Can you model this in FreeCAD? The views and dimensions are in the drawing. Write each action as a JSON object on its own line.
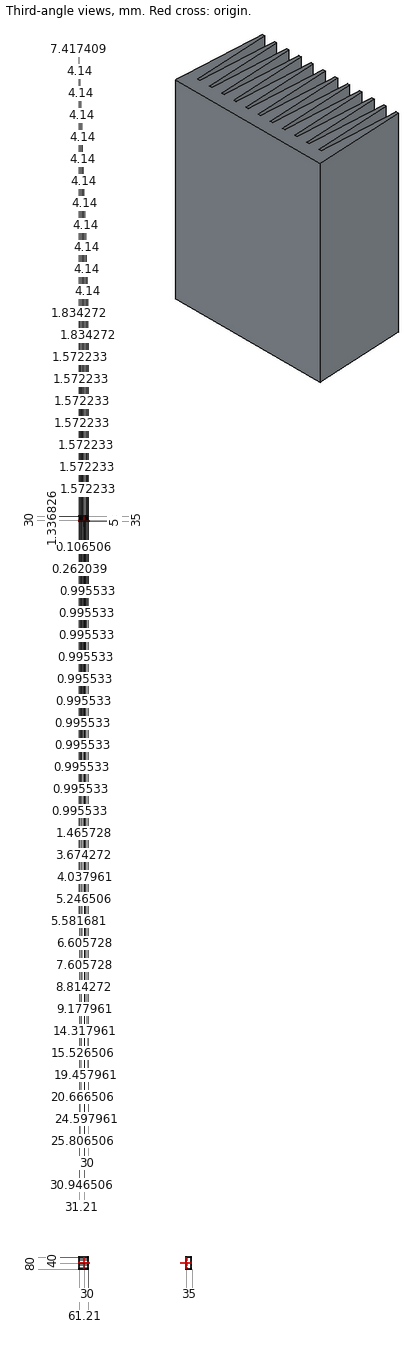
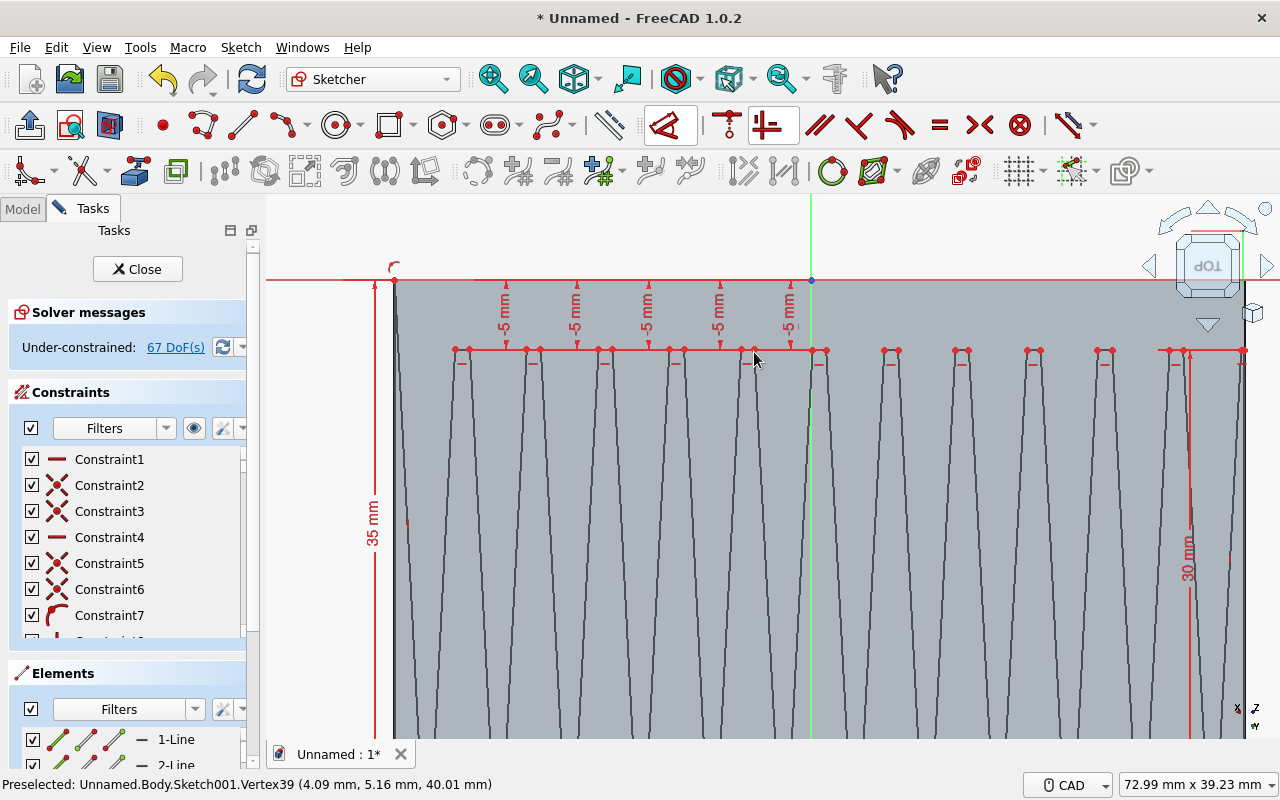
{"action": "left_click", "coordinate": [813, 350]}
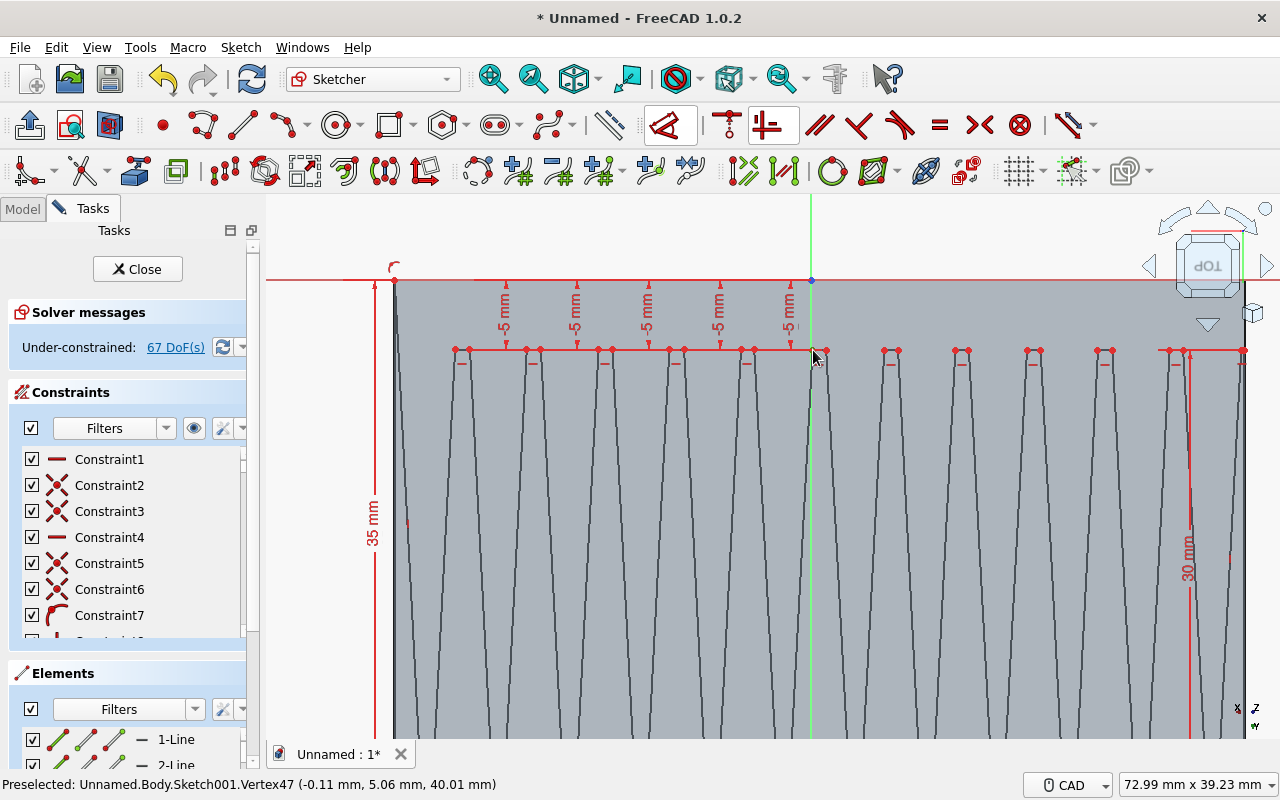
{"action": "left_click", "coordinate": [692, 126]}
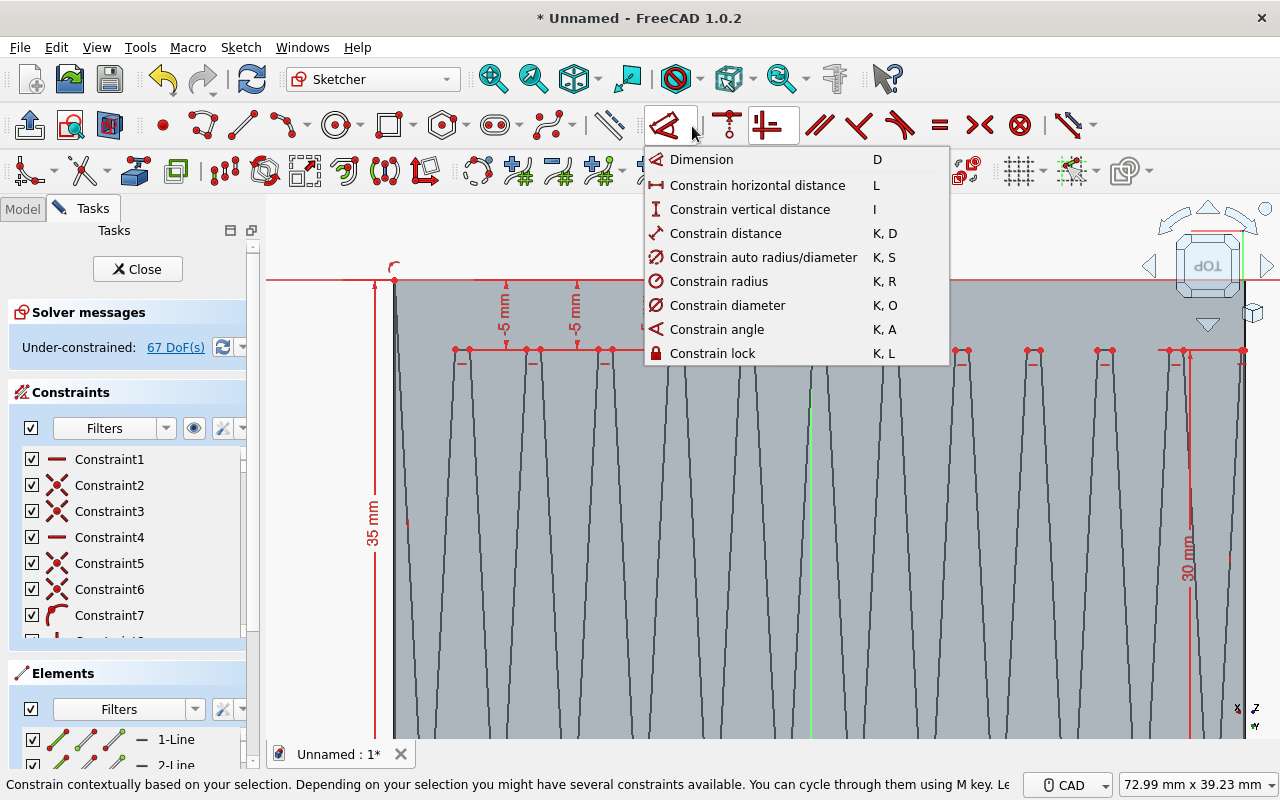
{"action": "left_click", "coordinate": [797, 209]}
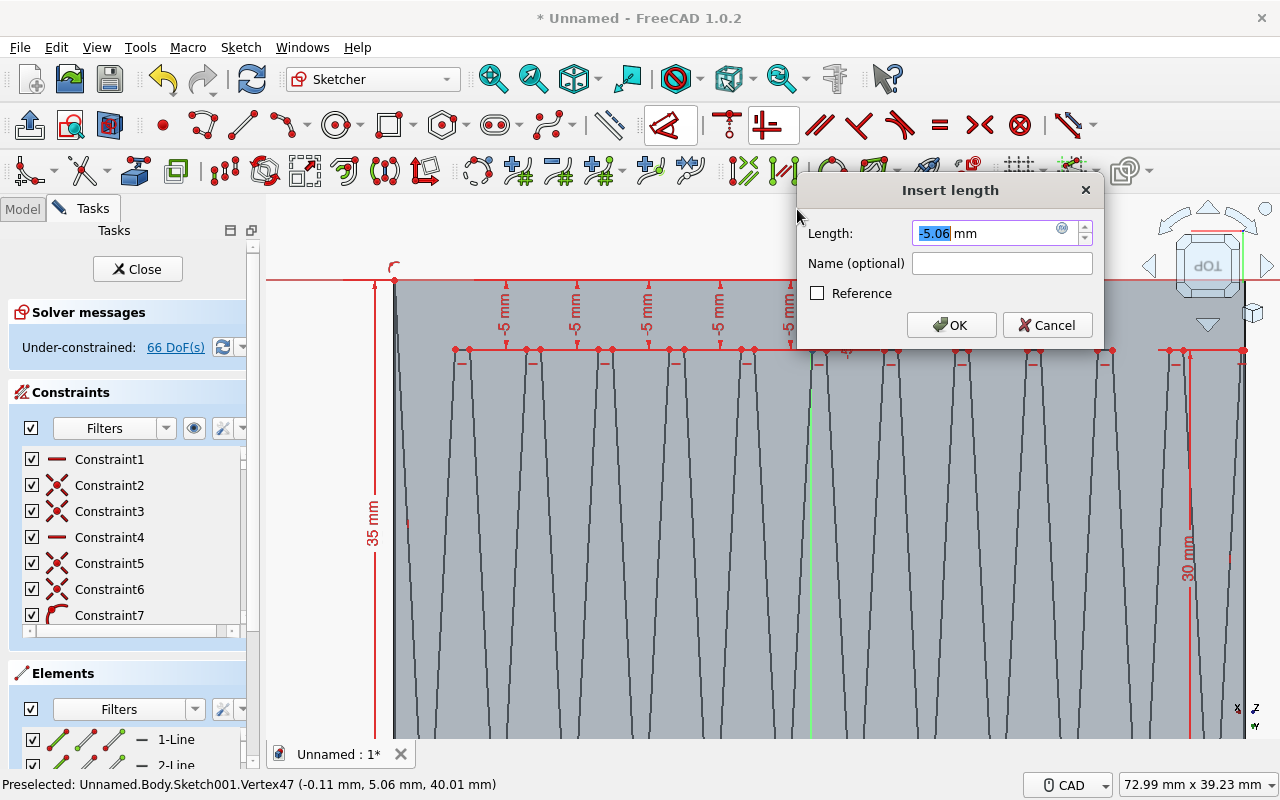
{"action": "type", "text": "-5"}
{"action": "key", "text": "Return"}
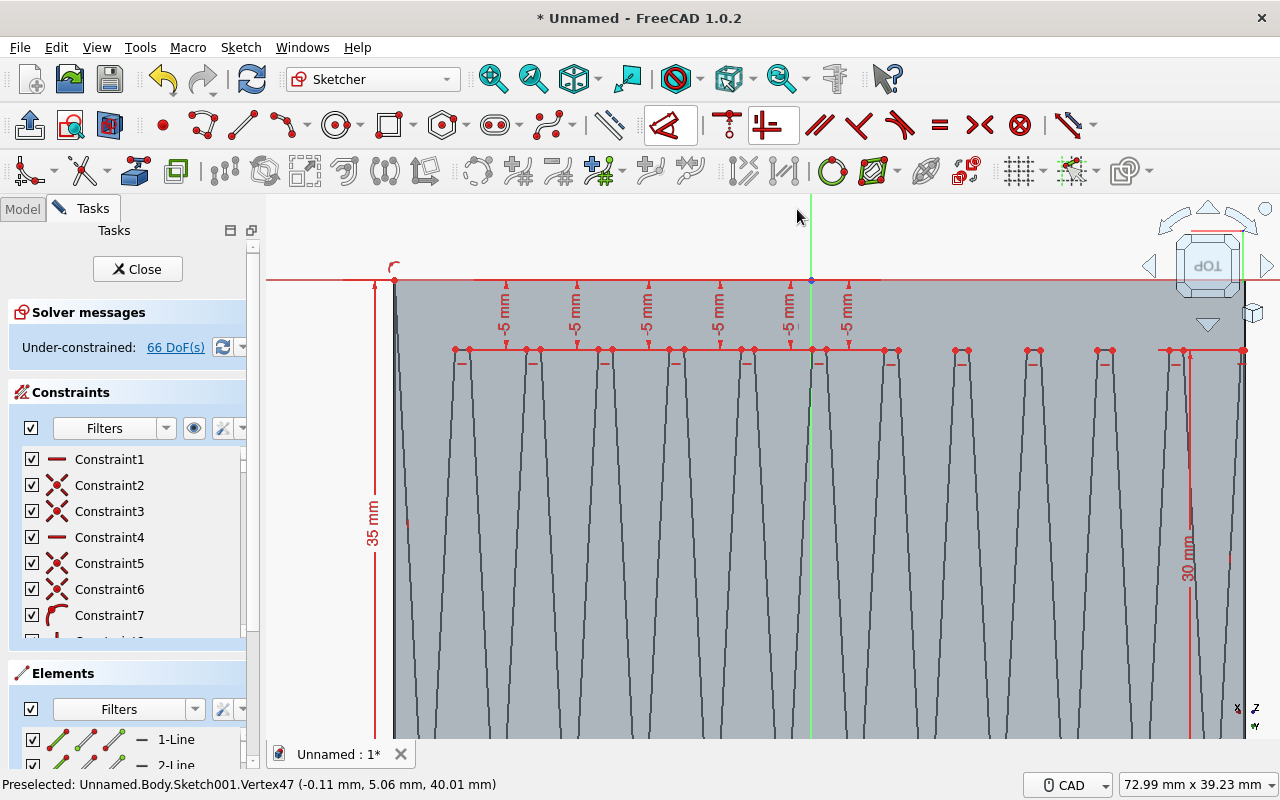
{"action": "left_click", "coordinate": [884, 350]}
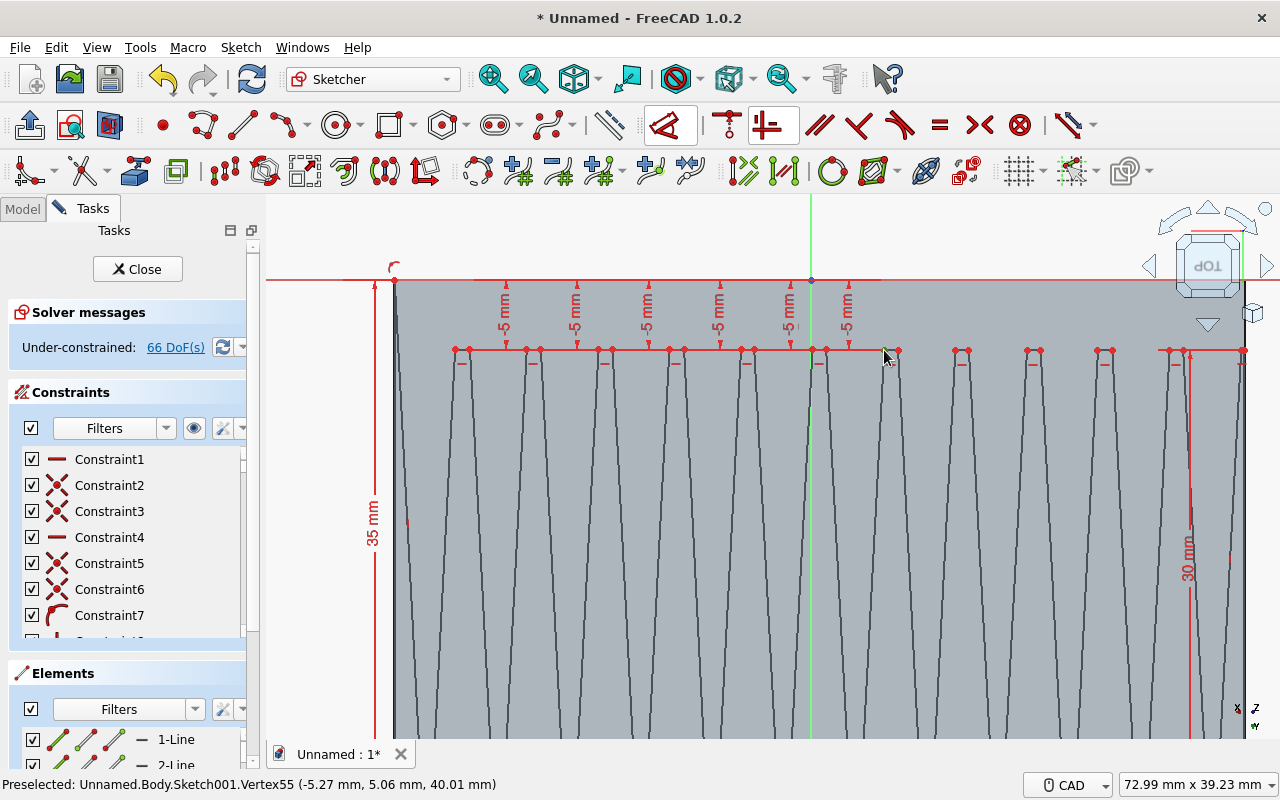
{"action": "key", "text": "i"}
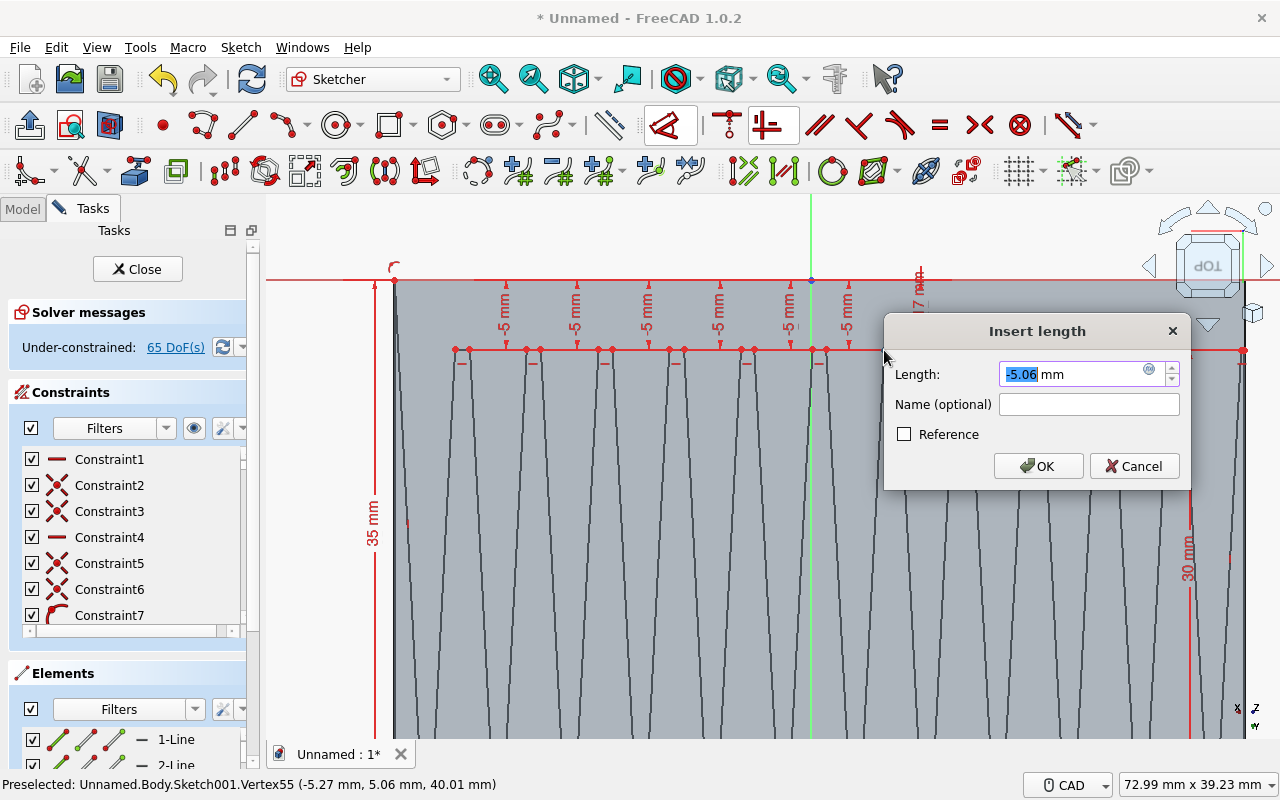
{"action": "type", "text": "-5"}
{"action": "key", "text": "Return"}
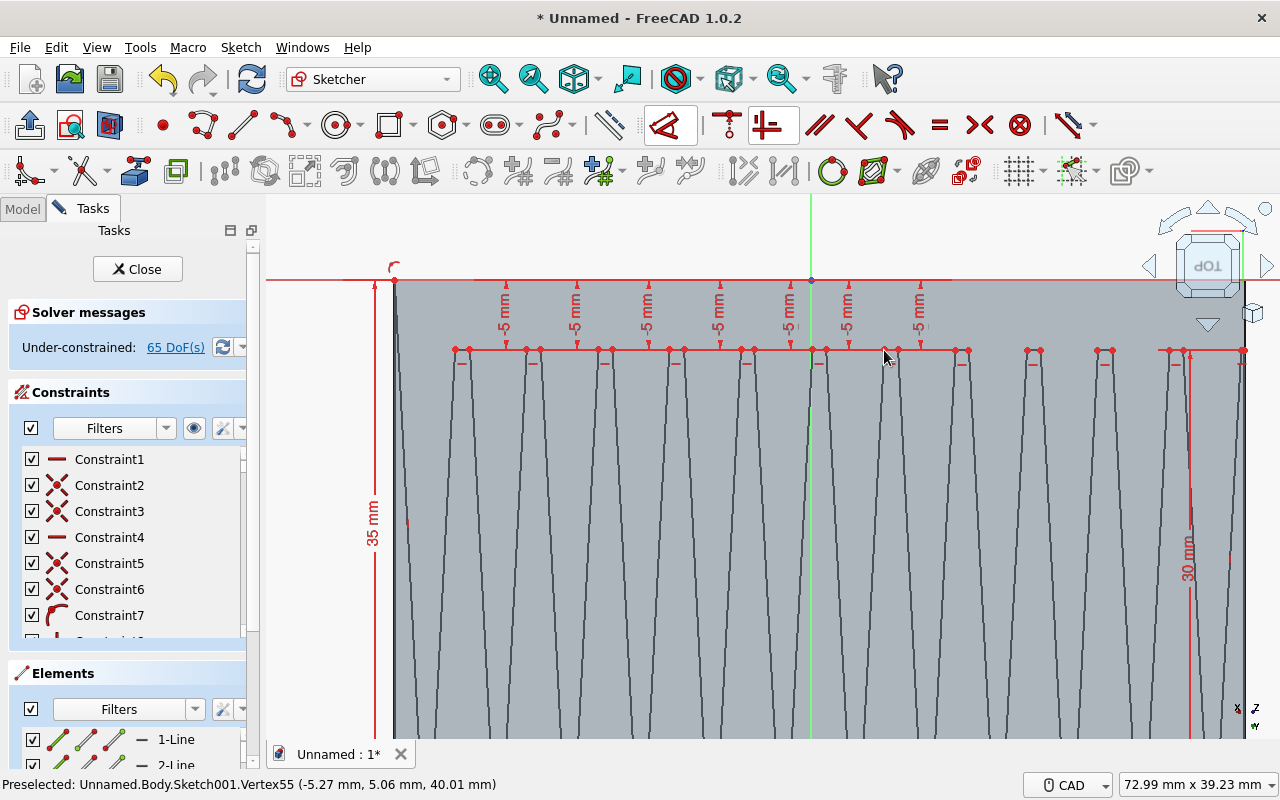
{"action": "left_click", "coordinate": [955, 350]}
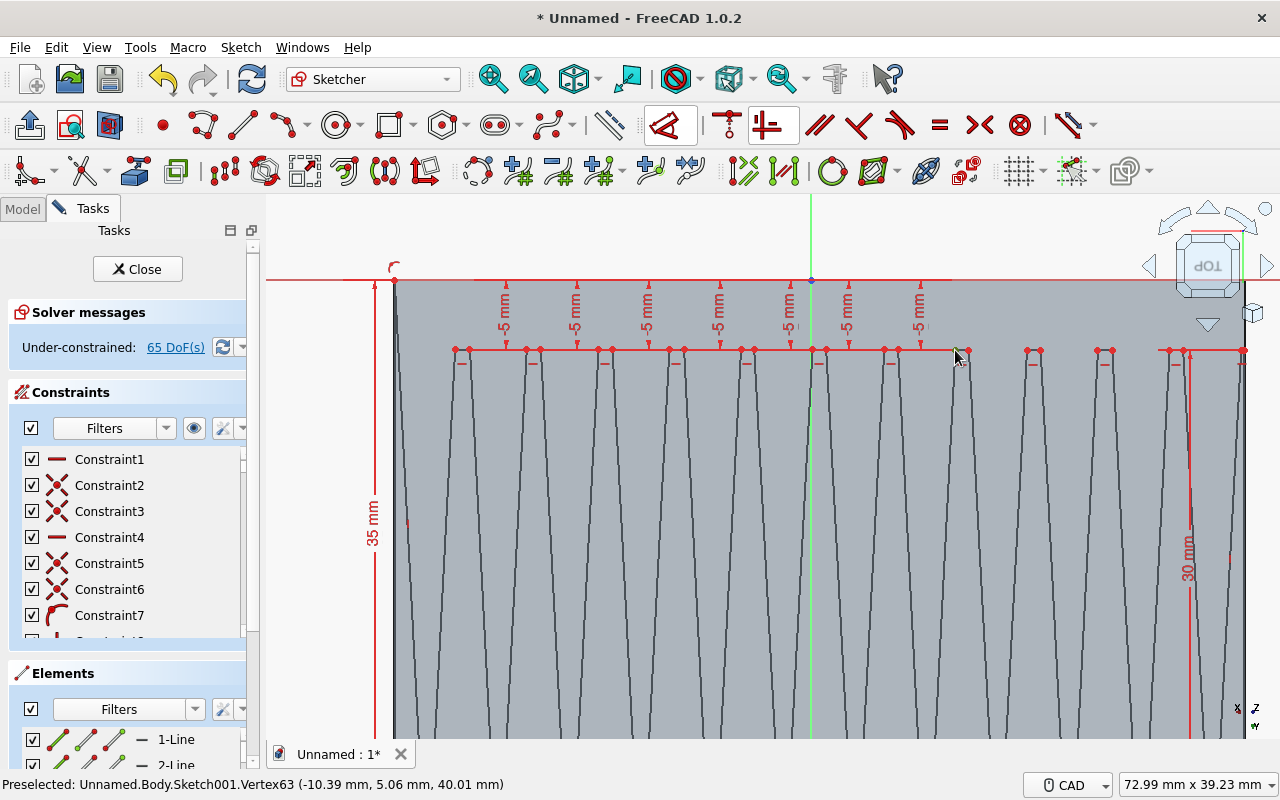
{"action": "left_click", "coordinate": [692, 126]}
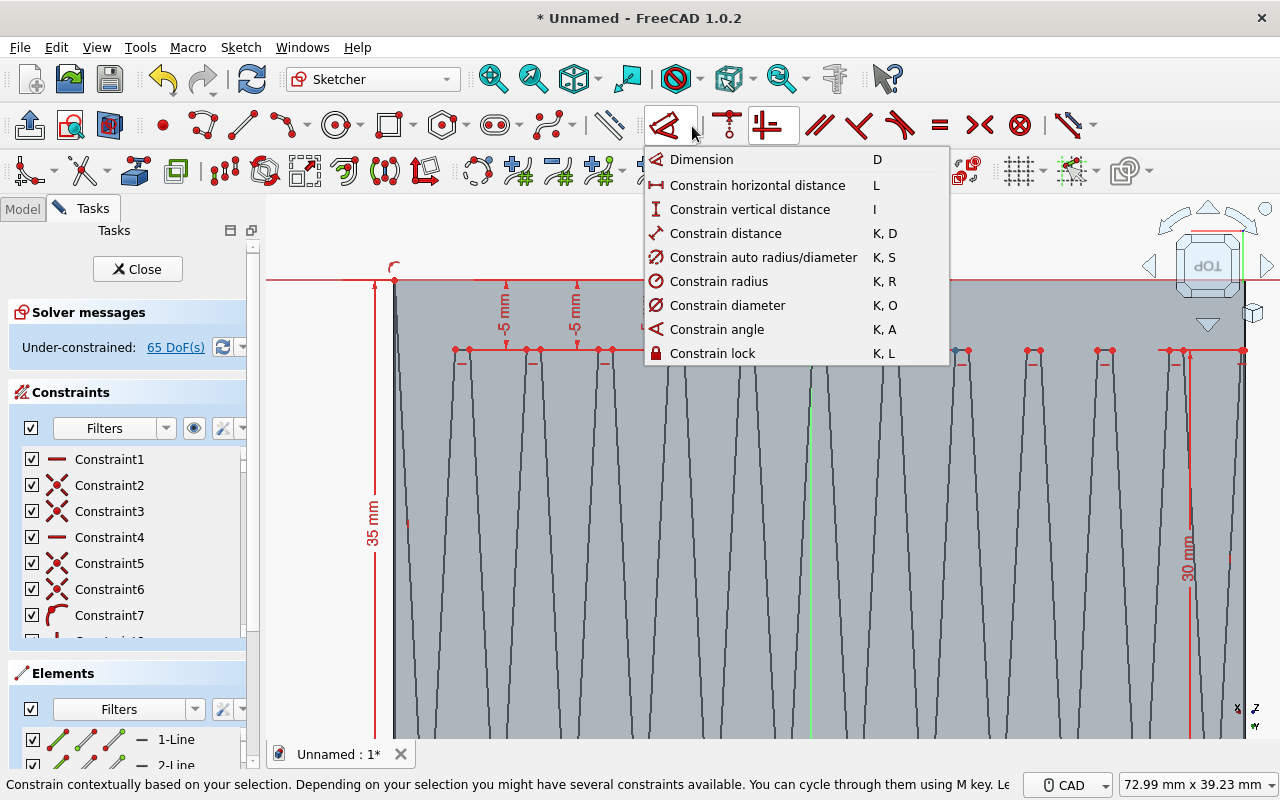
{"action": "left_click", "coordinate": [797, 209]}